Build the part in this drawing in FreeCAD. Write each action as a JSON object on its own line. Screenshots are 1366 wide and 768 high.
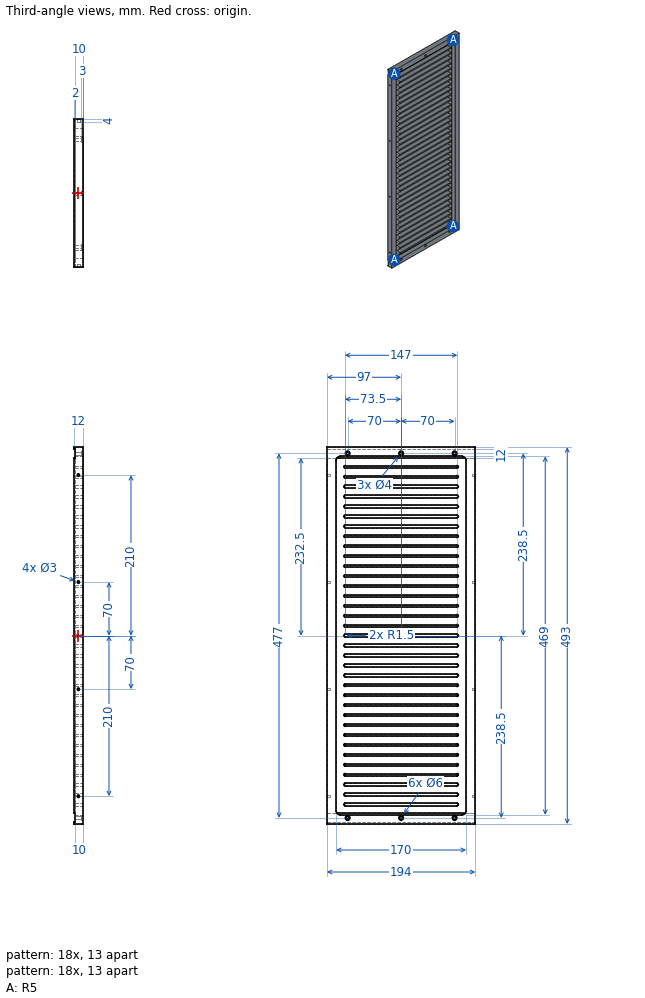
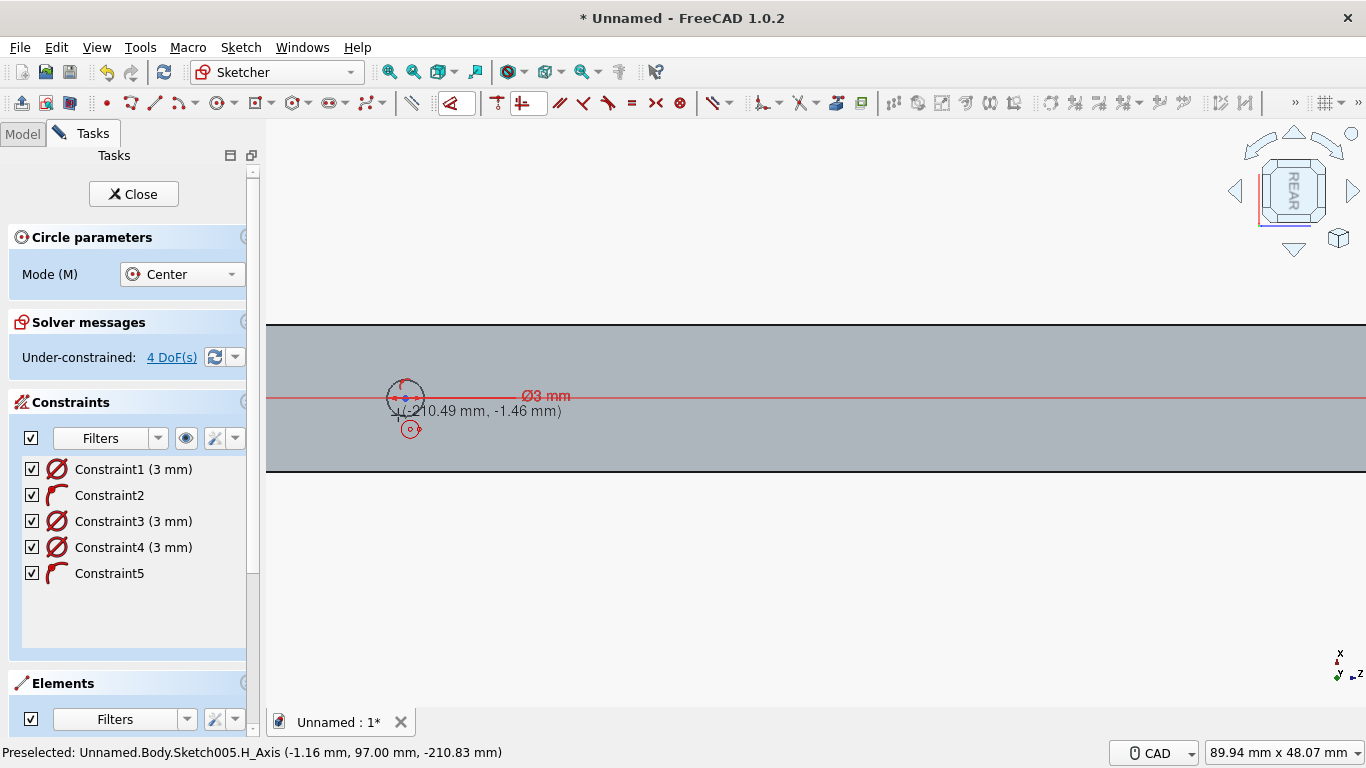
{"action": "scroll", "coordinate": [399, 415], "scroll_direction": "down", "scroll_amount": 10}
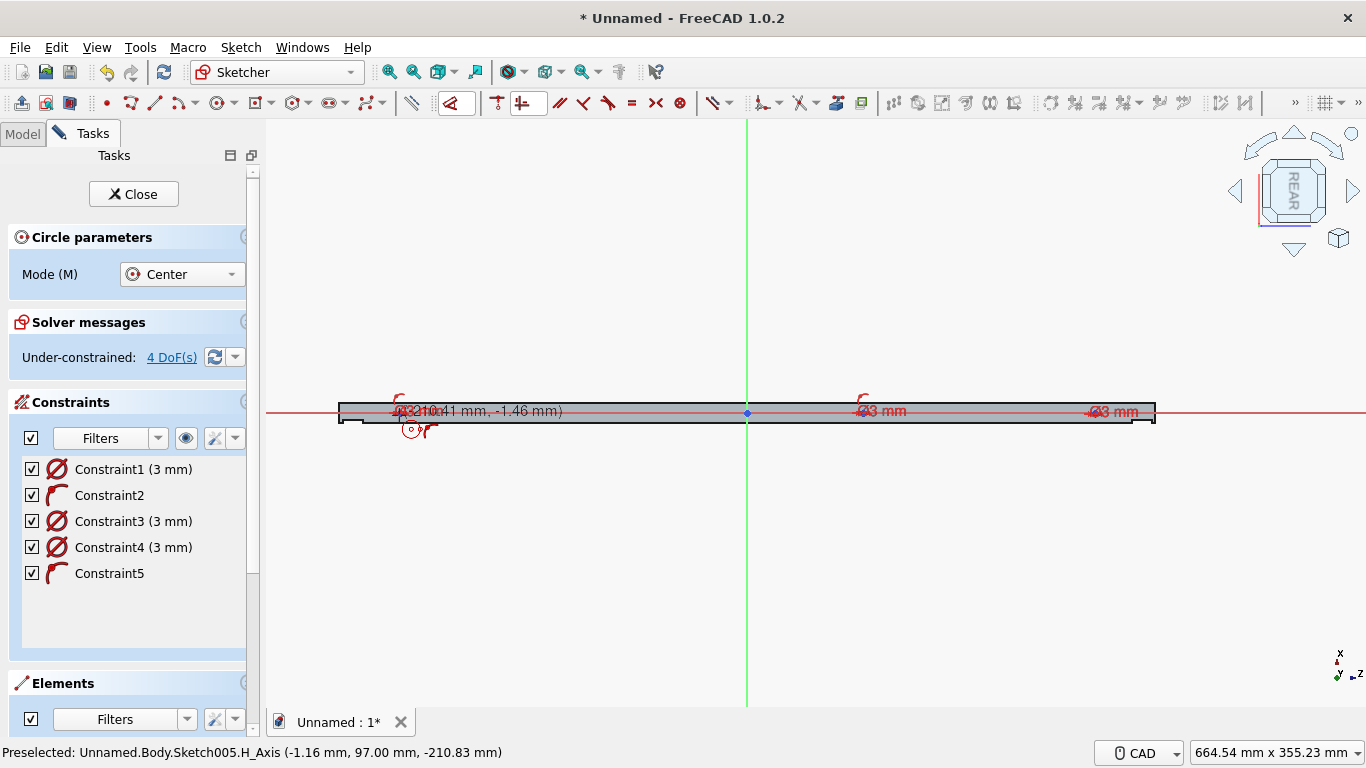
{"action": "scroll", "coordinate": [632, 413], "scroll_direction": "up", "scroll_amount": 12}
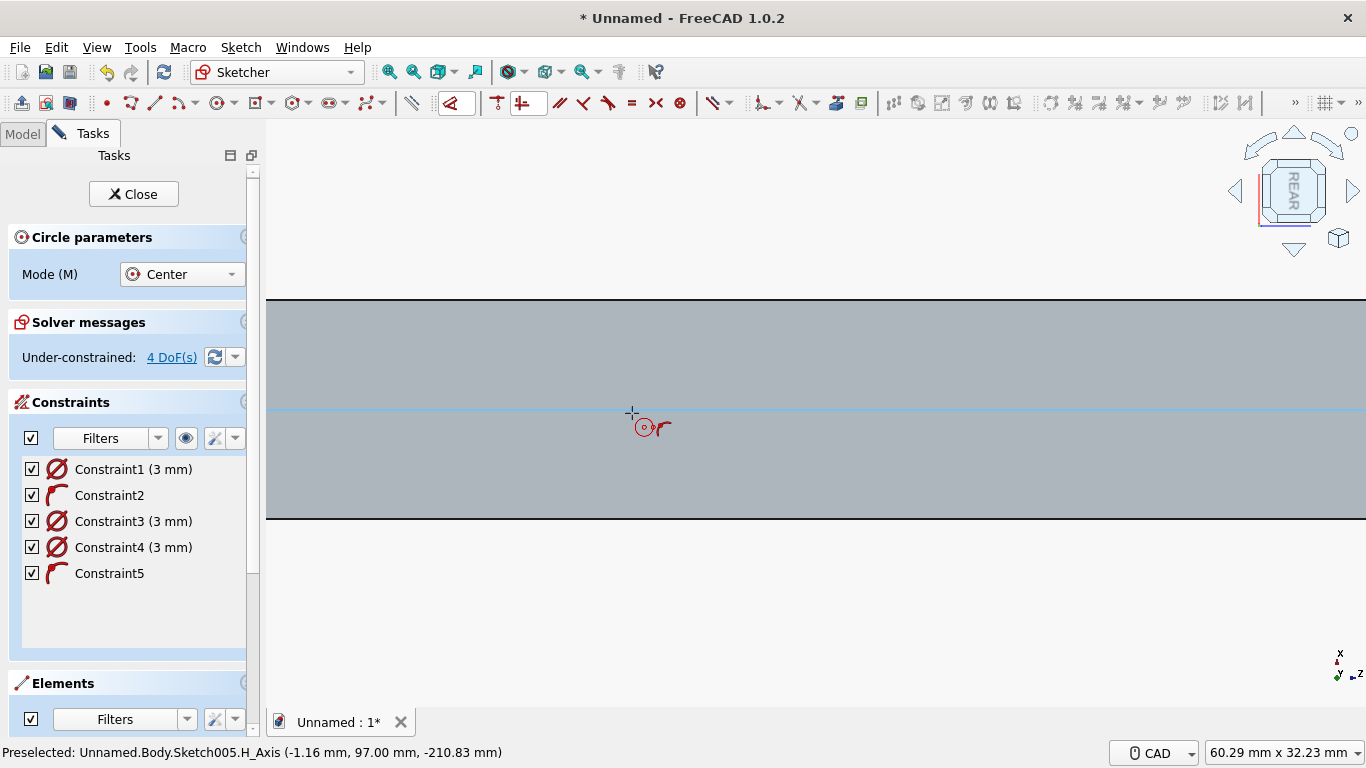
{"action": "scroll", "coordinate": [632, 413], "scroll_direction": "down", "scroll_amount": 12}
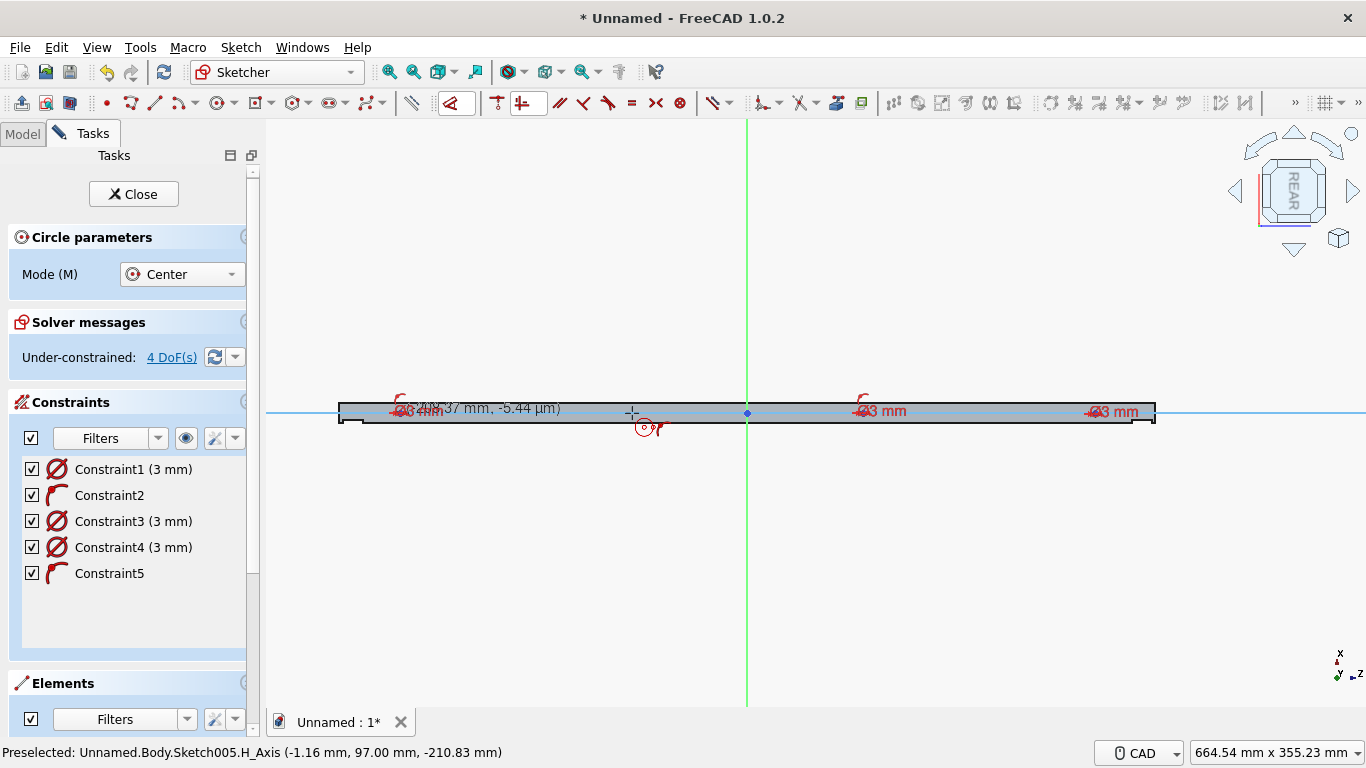
{"action": "left_click", "coordinate": [632, 413]}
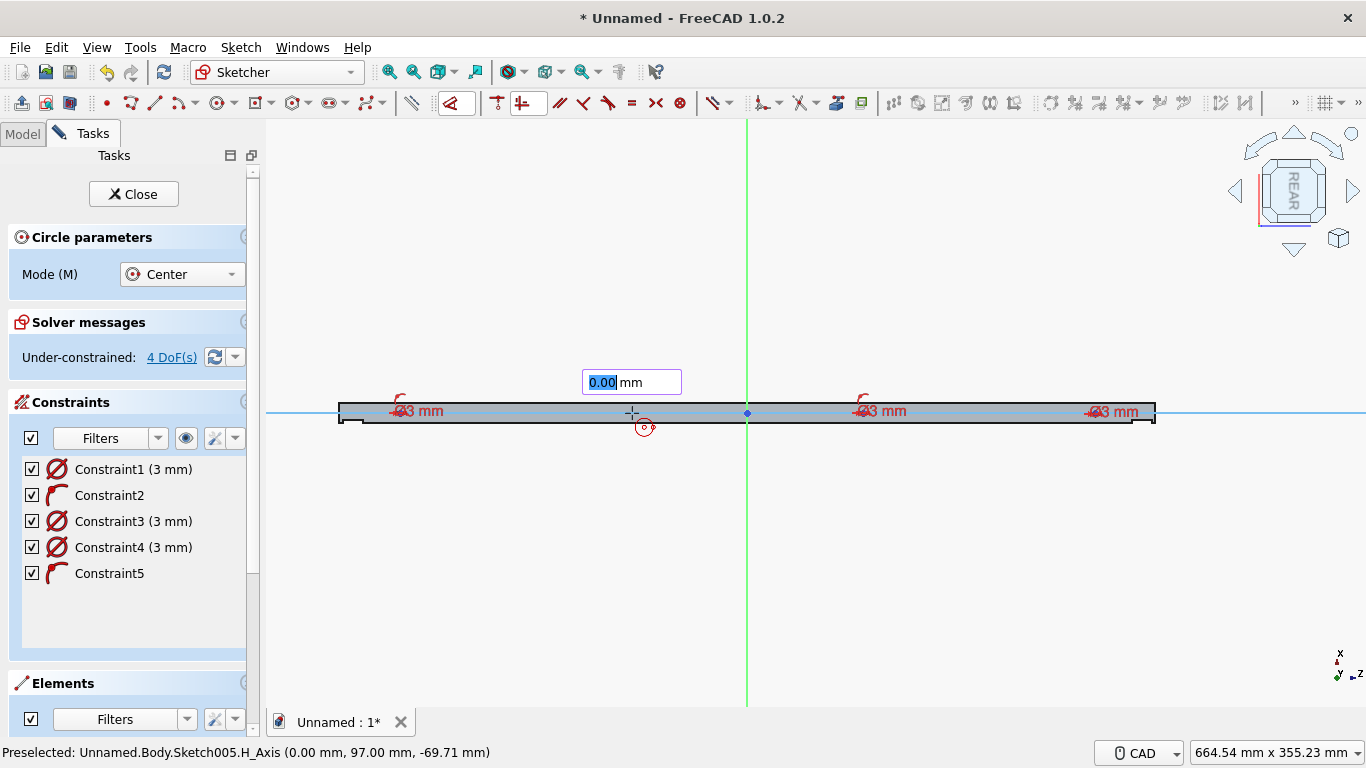
{"action": "scroll", "coordinate": [631, 415], "scroll_direction": "up", "scroll_amount": 10}
{"action": "mouse_move", "coordinate": [626, 415]}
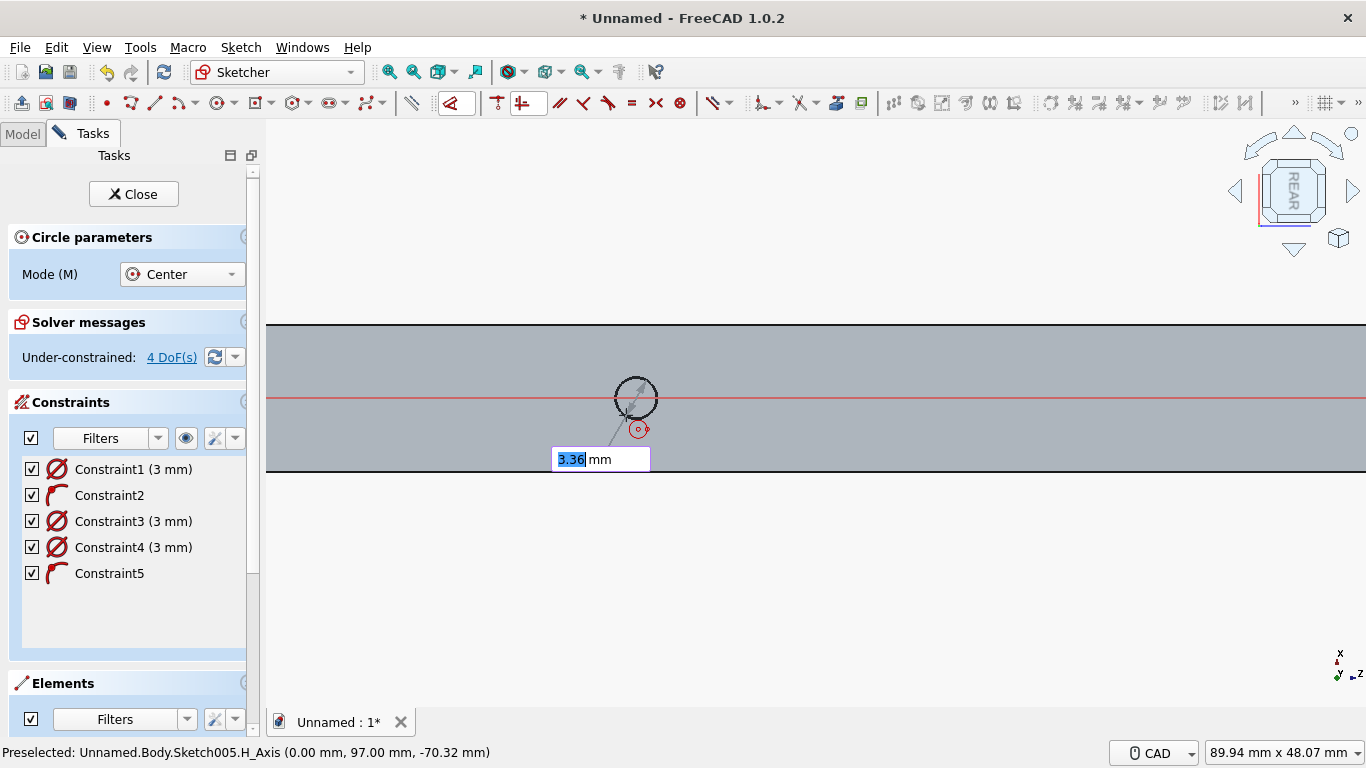
{"action": "type", "text": "3"}
{"action": "key", "text": "Return"}
{"action": "key", "text": "Escape"}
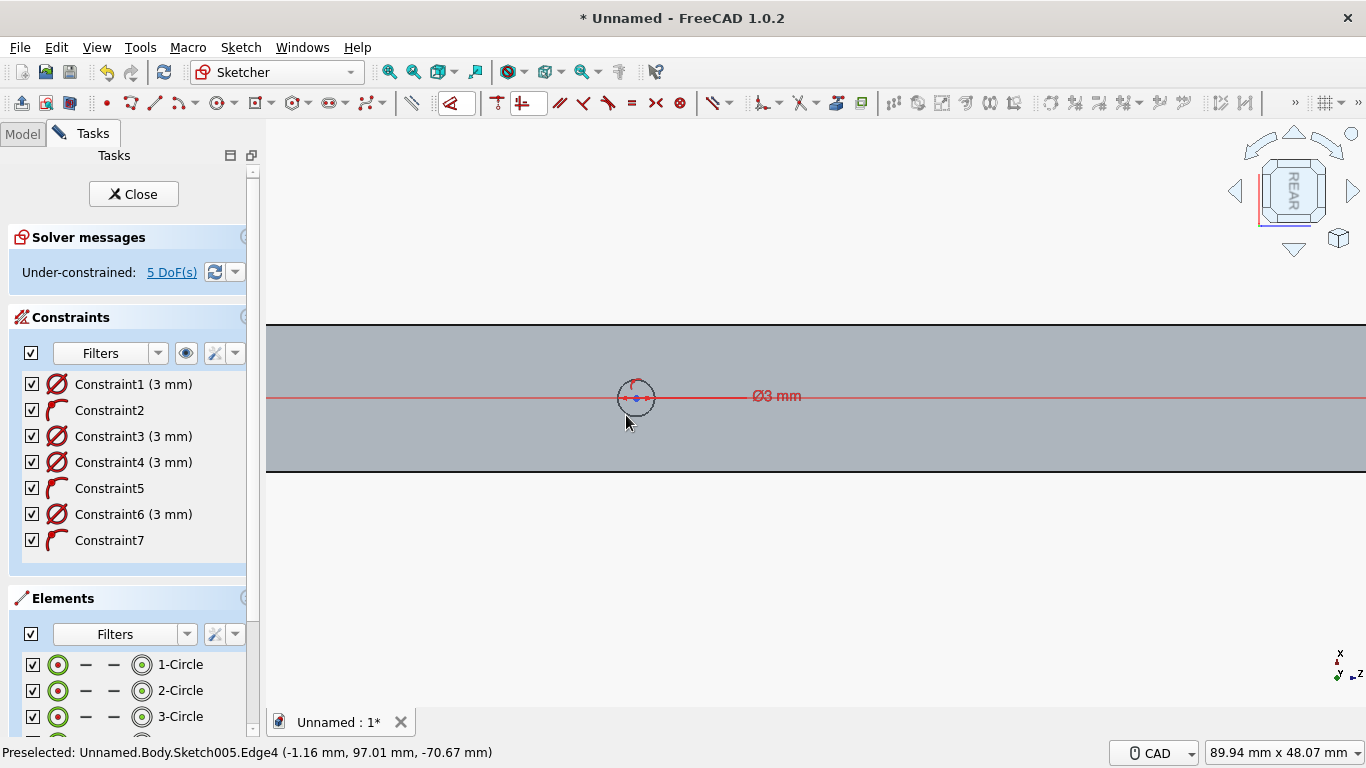
{"action": "scroll", "coordinate": [631, 415], "scroll_direction": "down", "scroll_amount": 10}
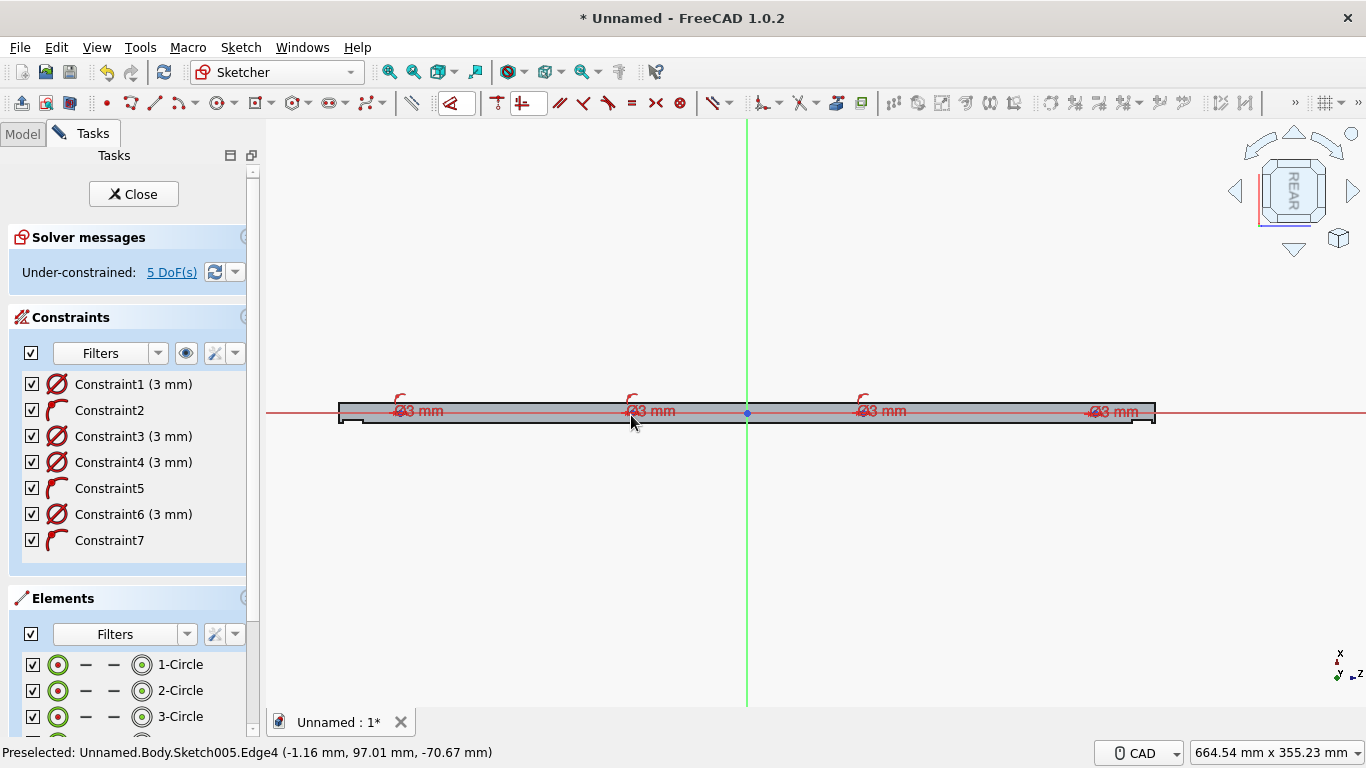
{"action": "left_click", "coordinate": [1095, 414]}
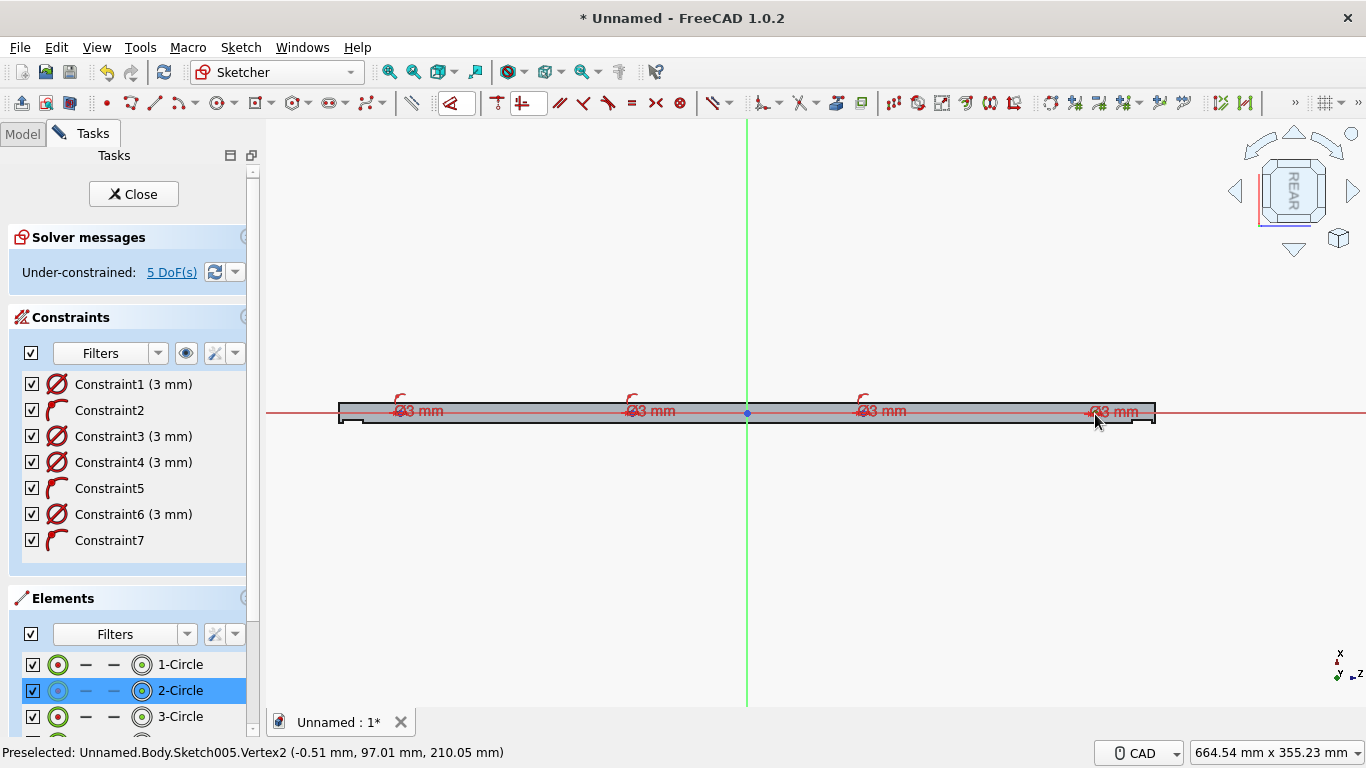
{"action": "left_click", "coordinate": [359, 413]}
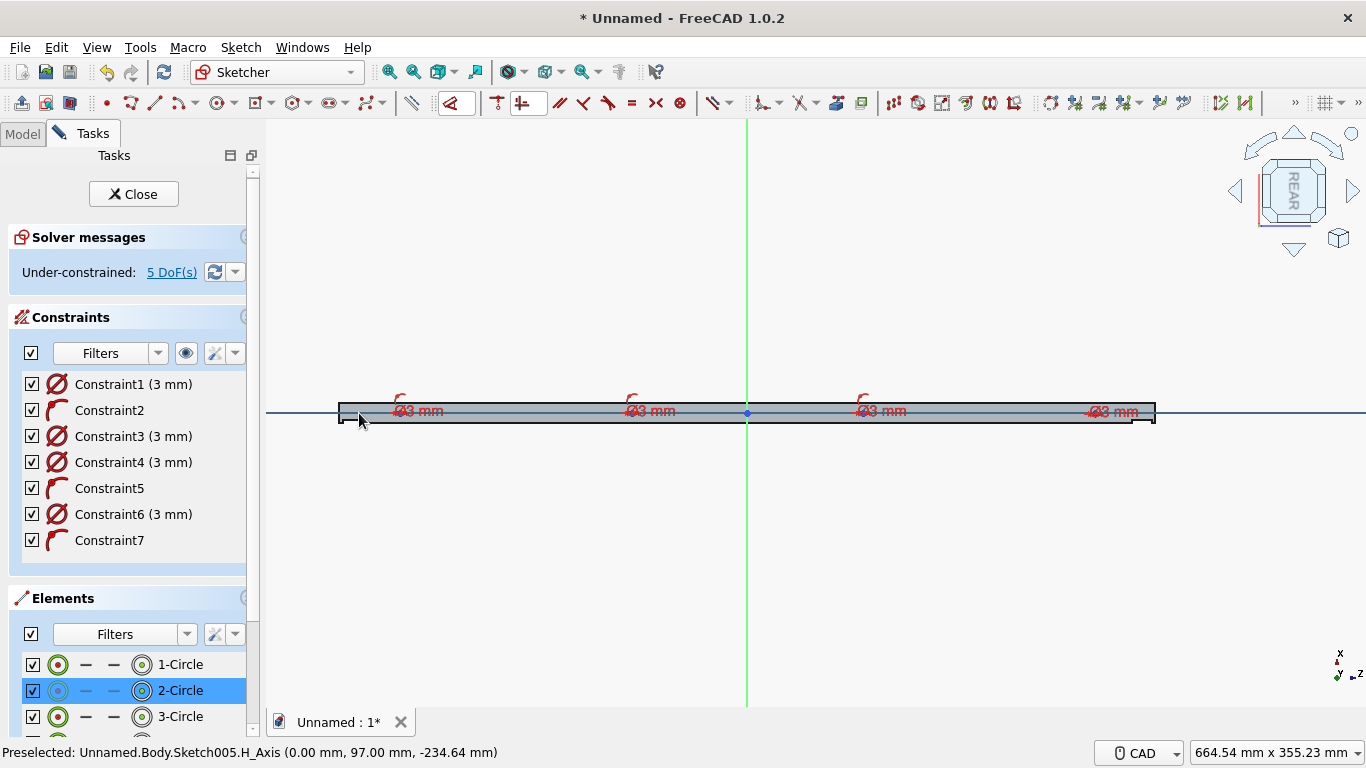
{"action": "left_click", "coordinate": [498, 104]}